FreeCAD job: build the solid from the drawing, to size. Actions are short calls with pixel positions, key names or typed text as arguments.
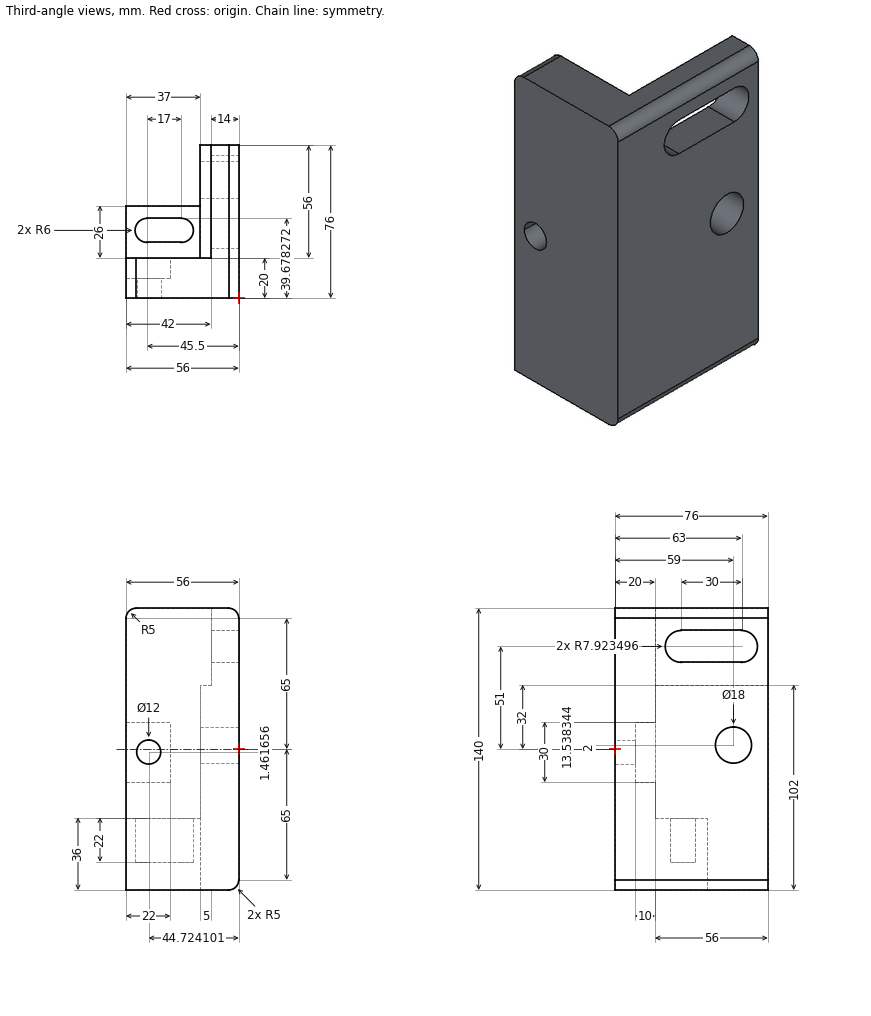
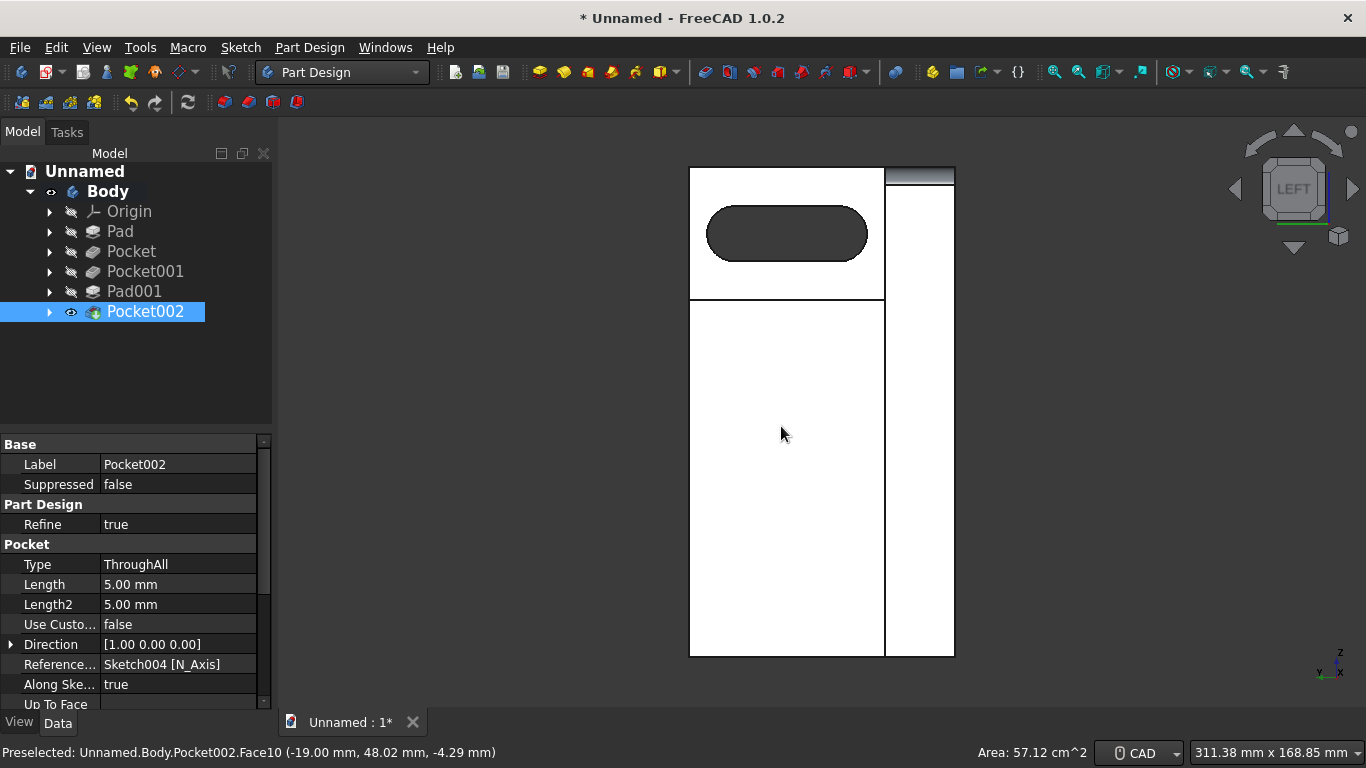
click(46, 72)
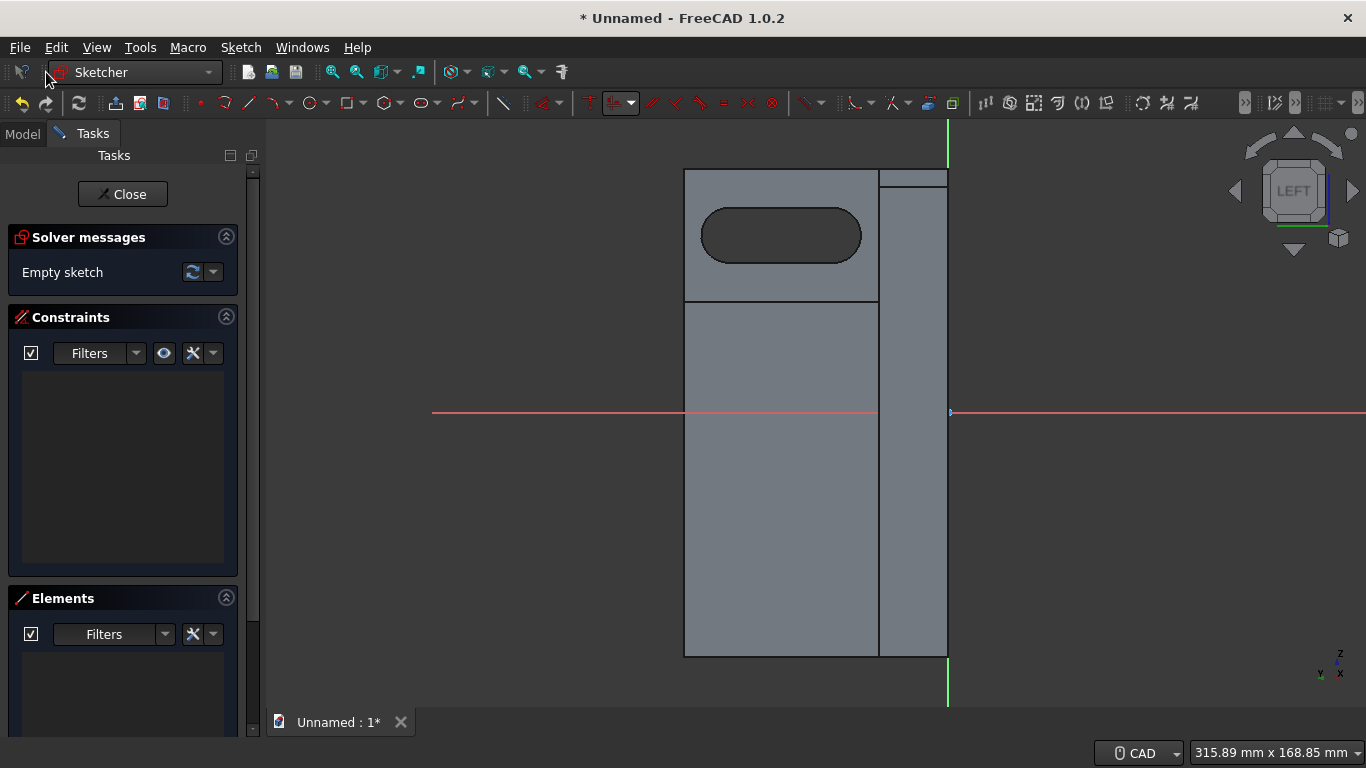
scroll(742, 405, up, 9)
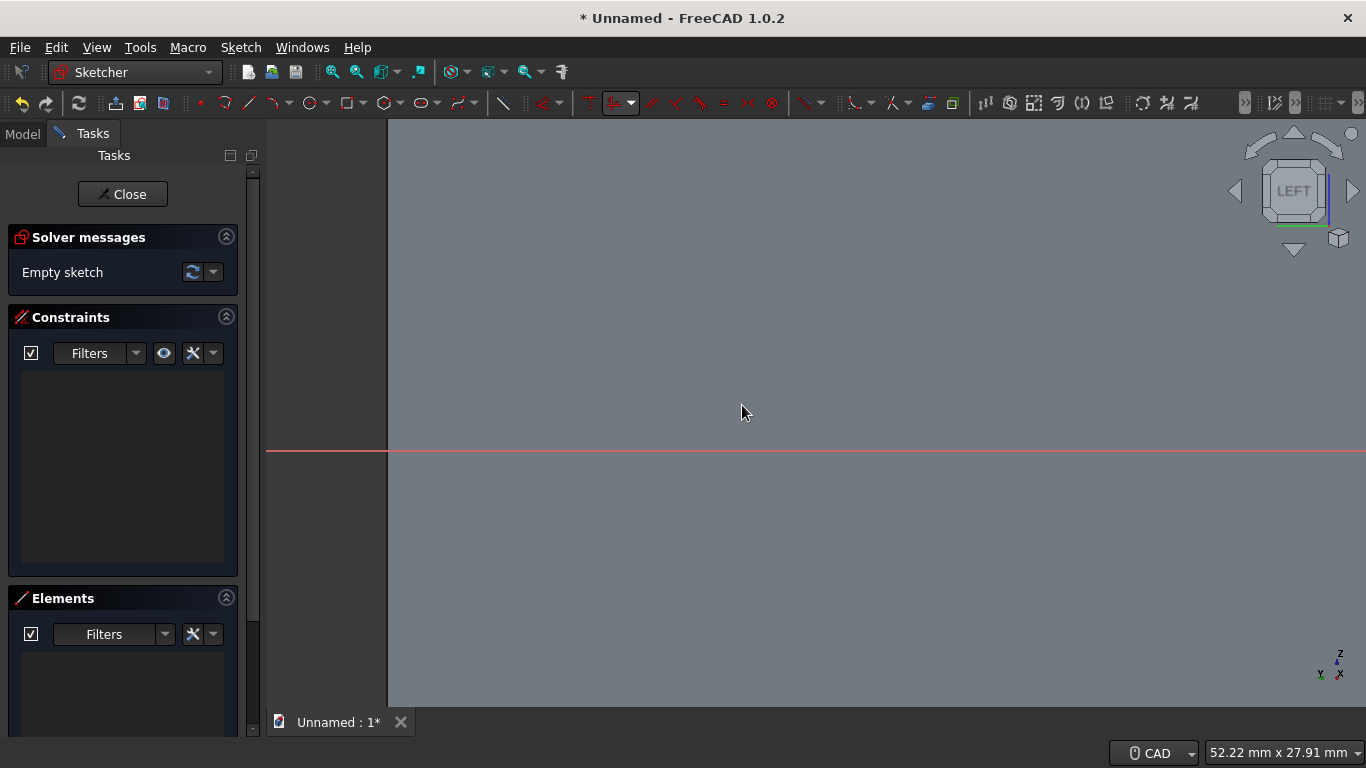
click(310, 104)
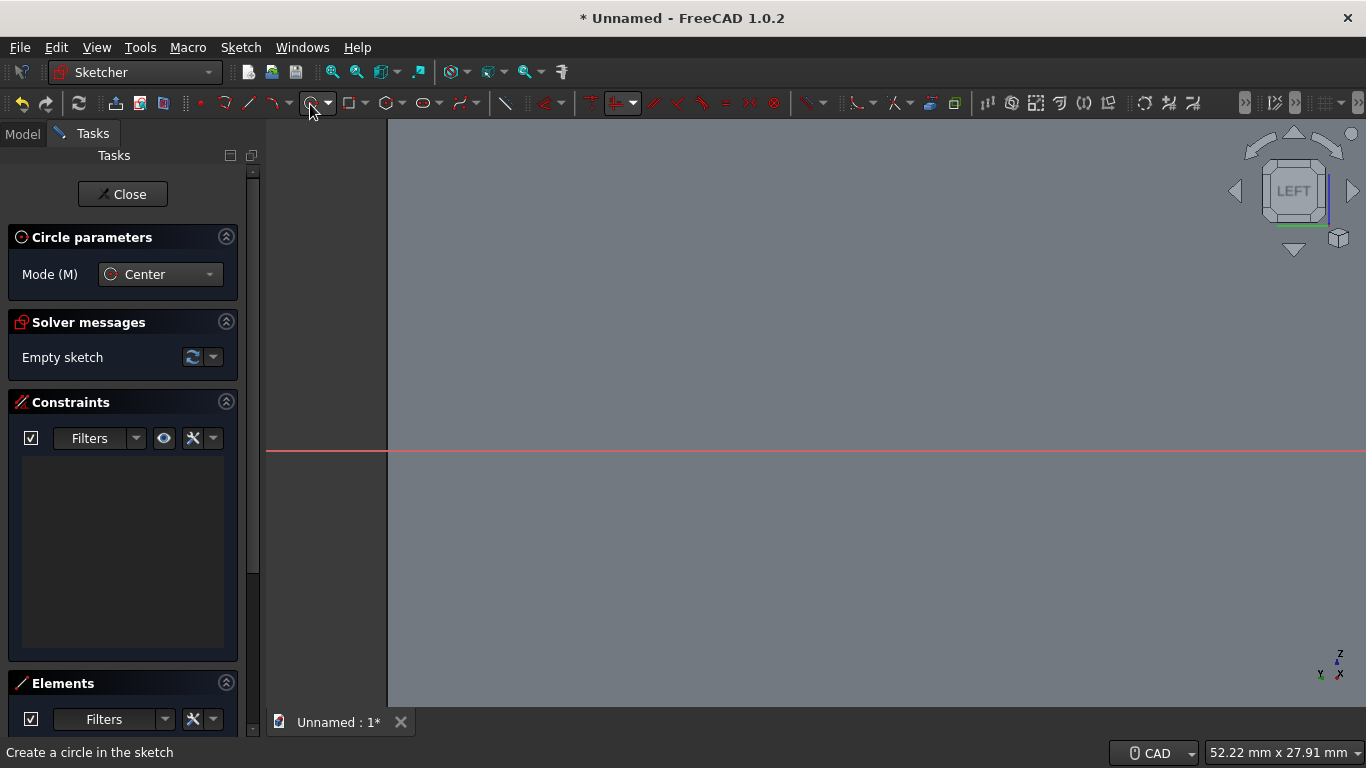
click(745, 409)
click(879, 275)
key(Escape)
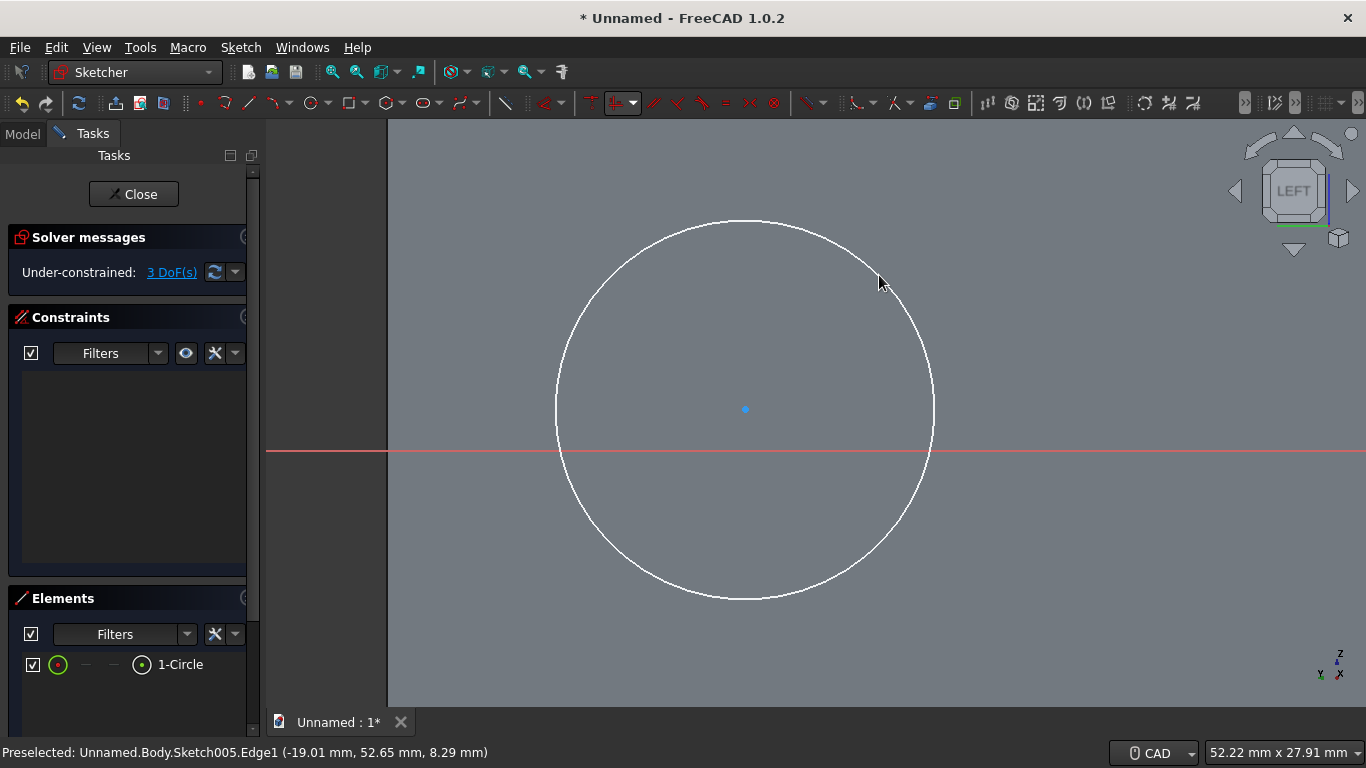
click(544, 104)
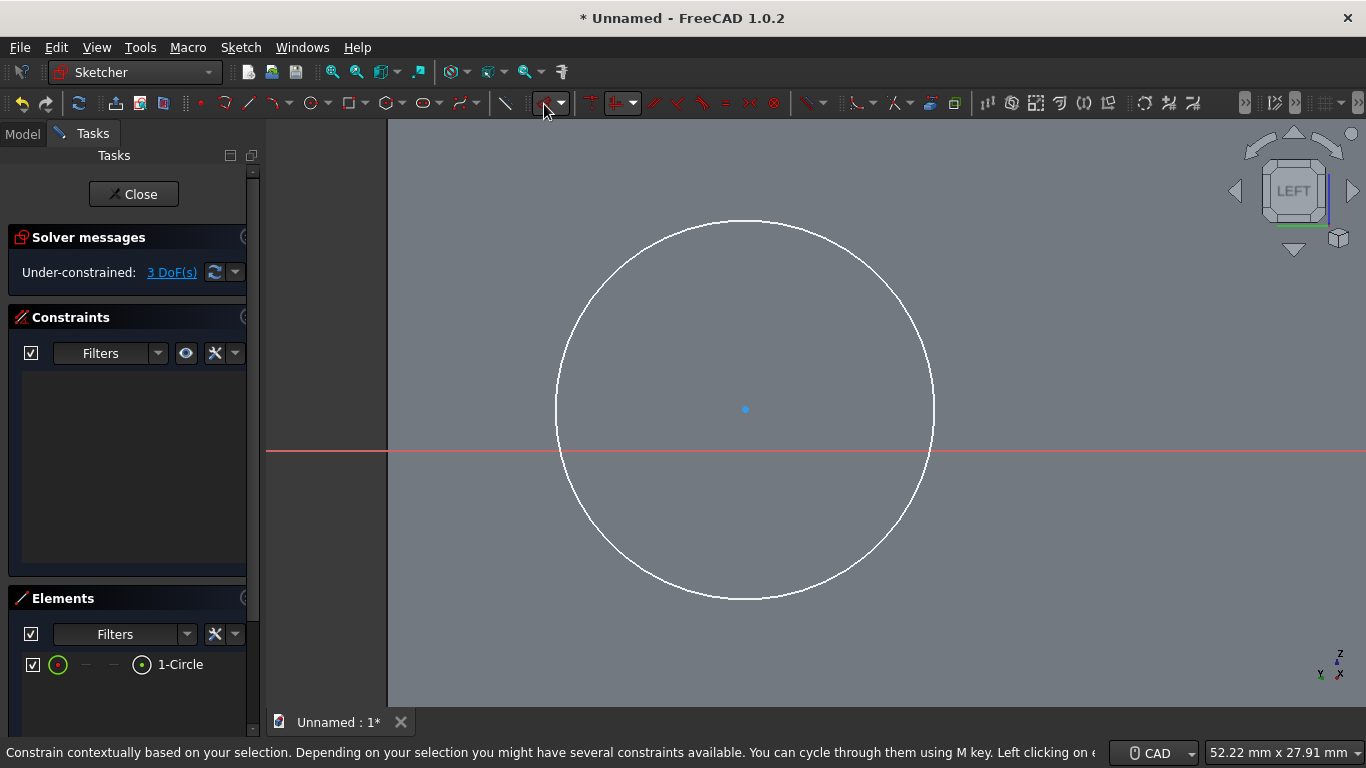
click(879, 276)
click(902, 253)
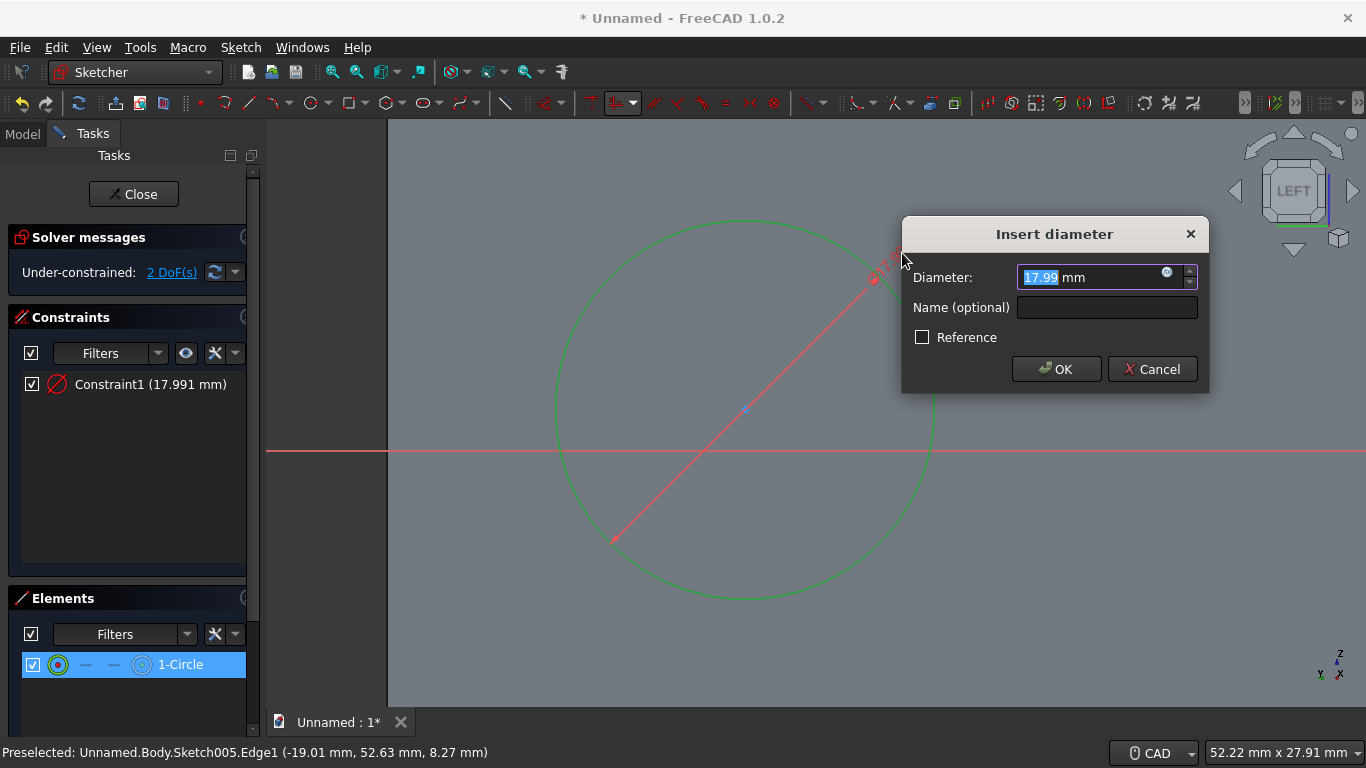
text(18)
key(Return)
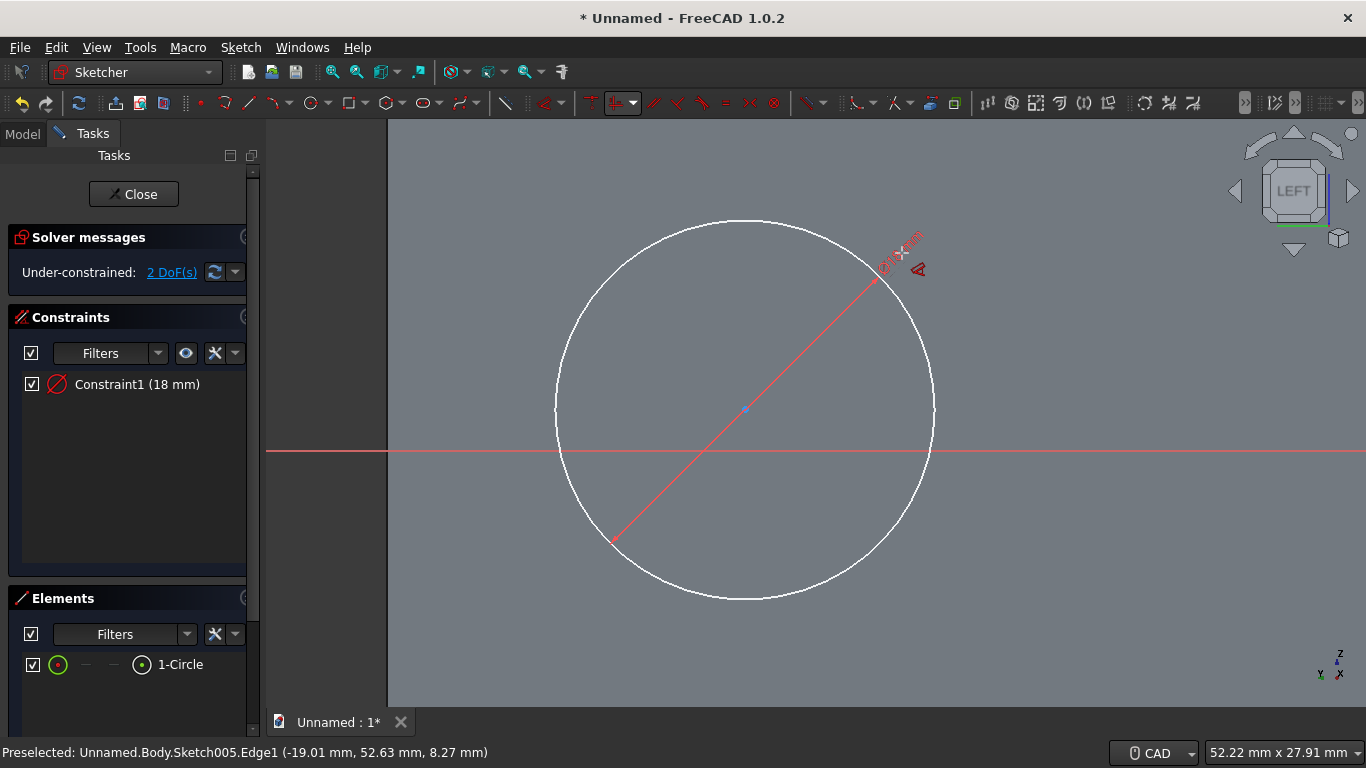
click(745, 410)
click(711, 430)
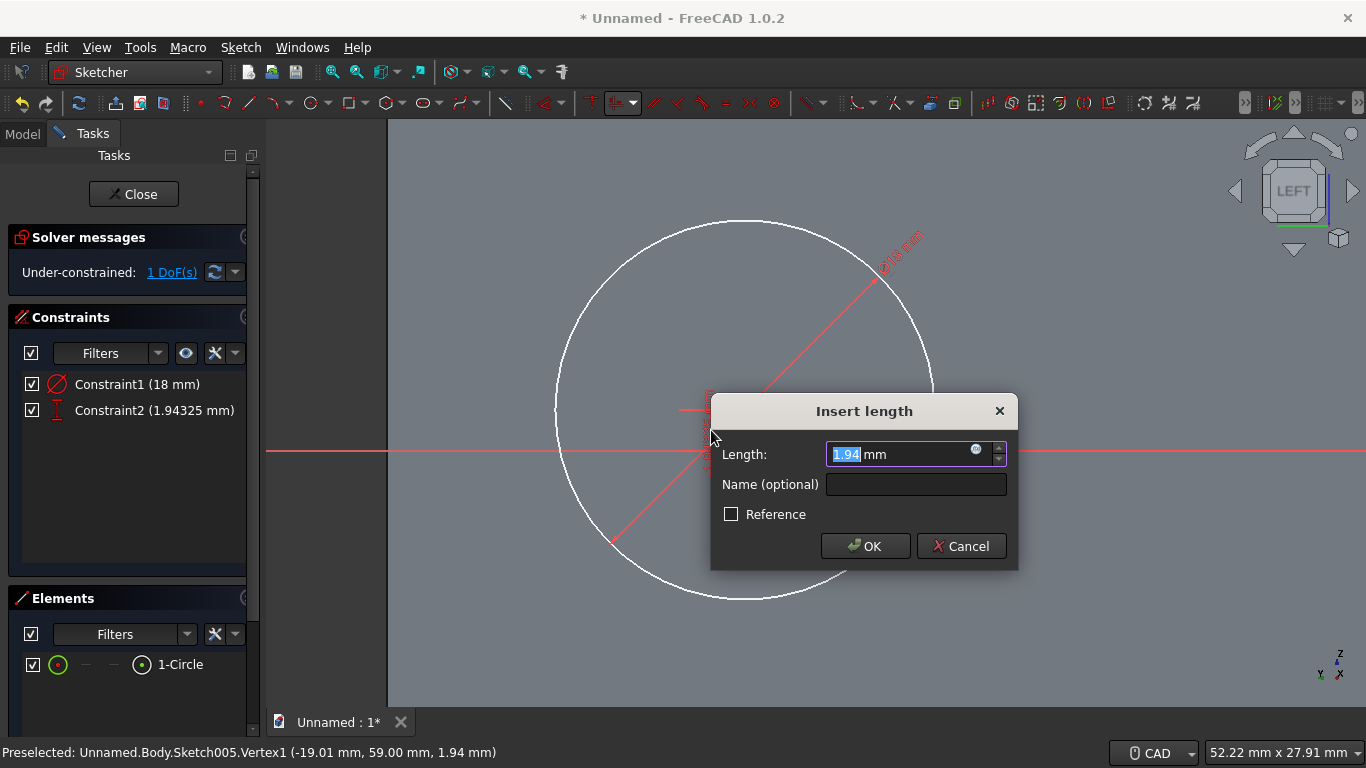
text(2)
key(Return)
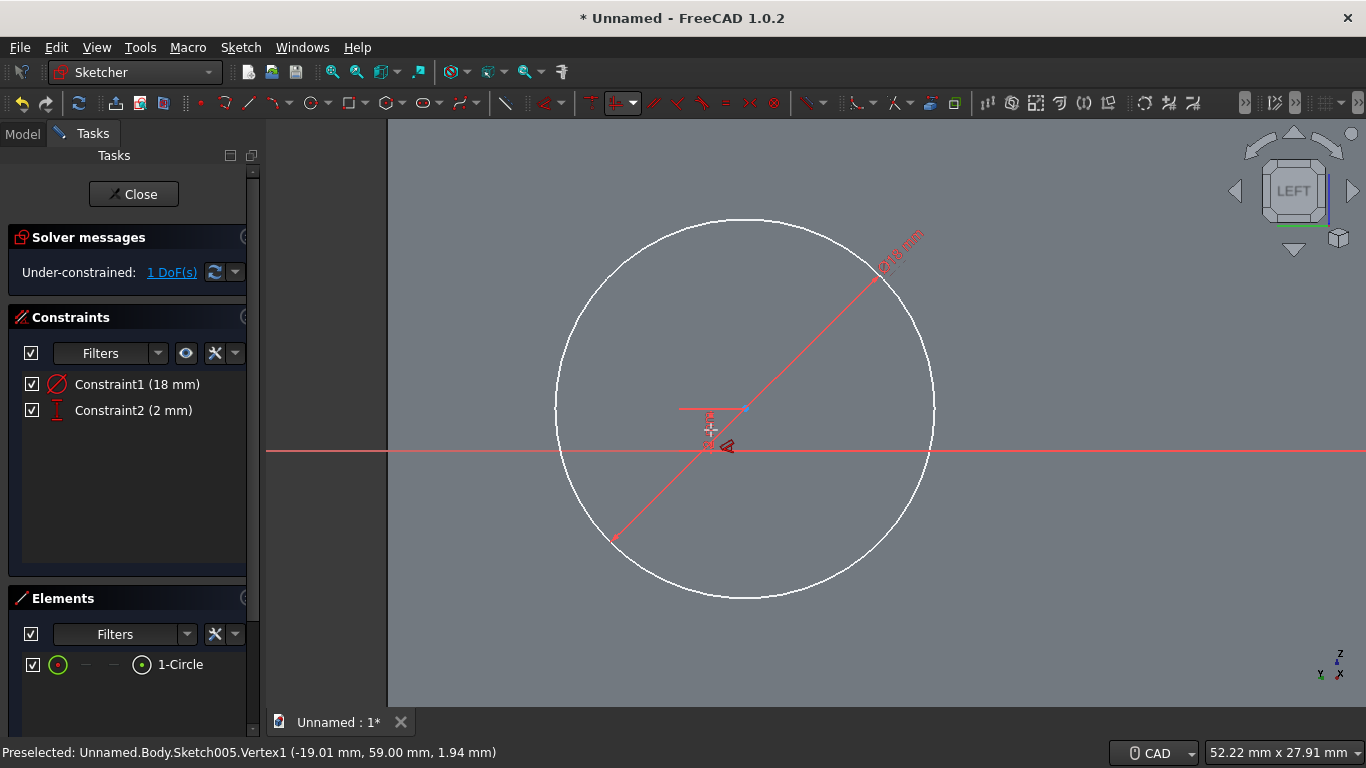
click(745, 409)
click(973, 485)